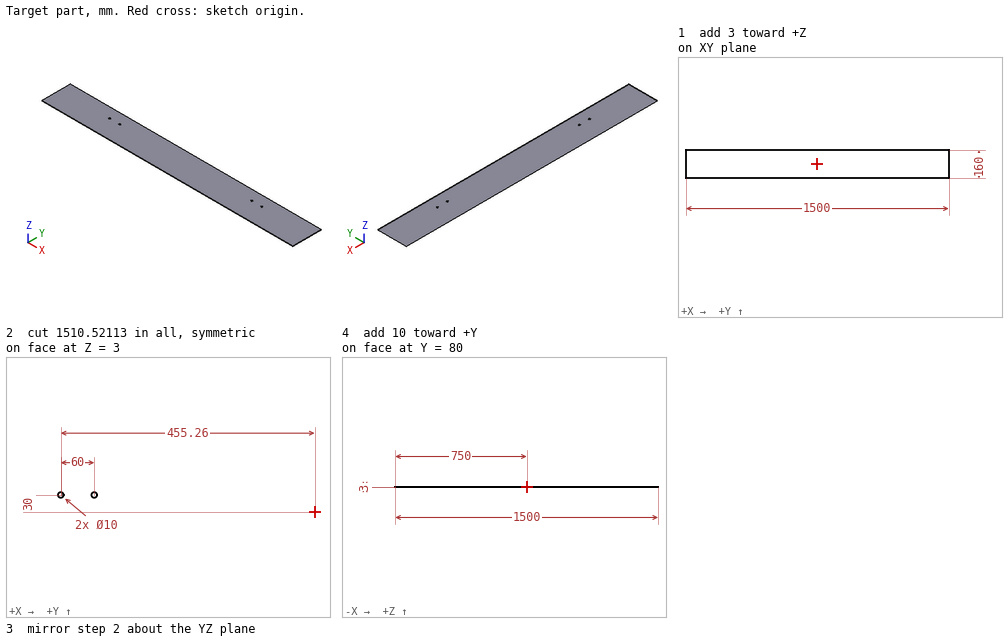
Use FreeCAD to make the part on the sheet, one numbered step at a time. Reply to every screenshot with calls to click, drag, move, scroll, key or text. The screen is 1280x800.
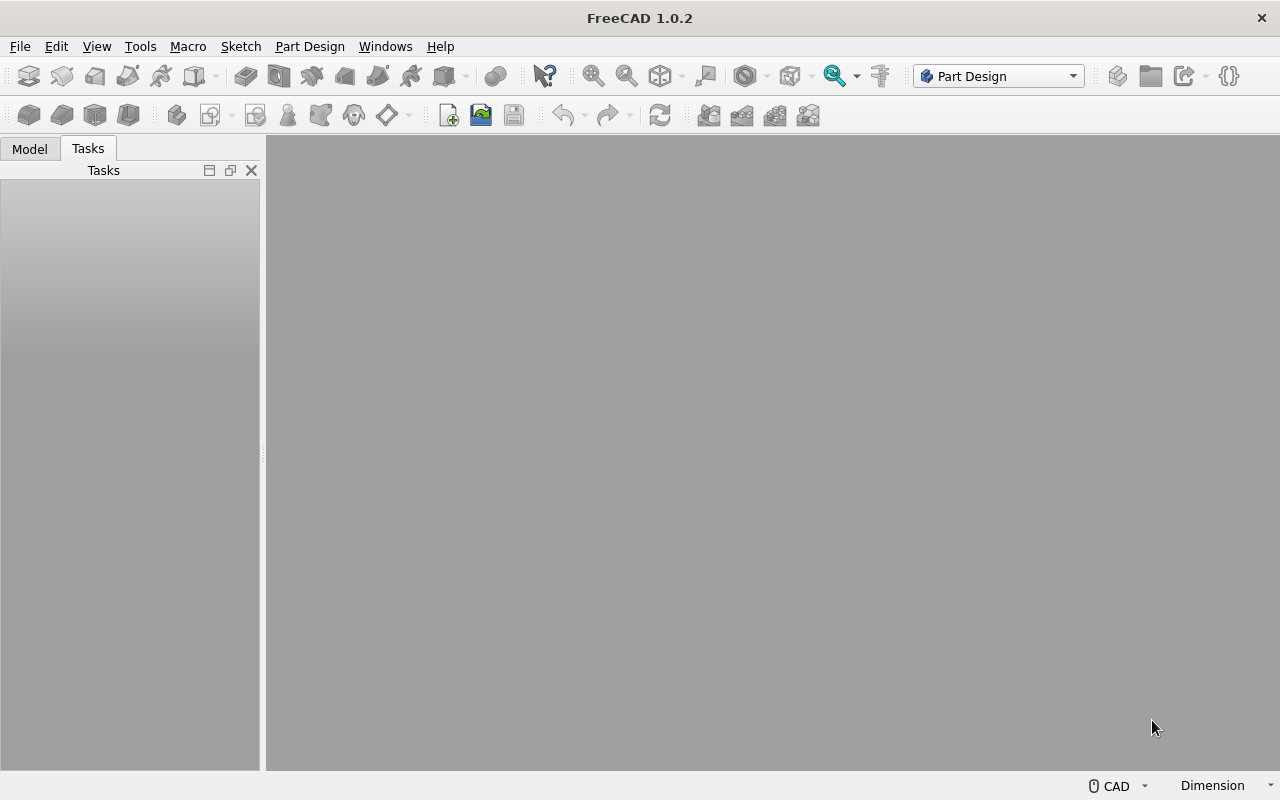
click(448, 116)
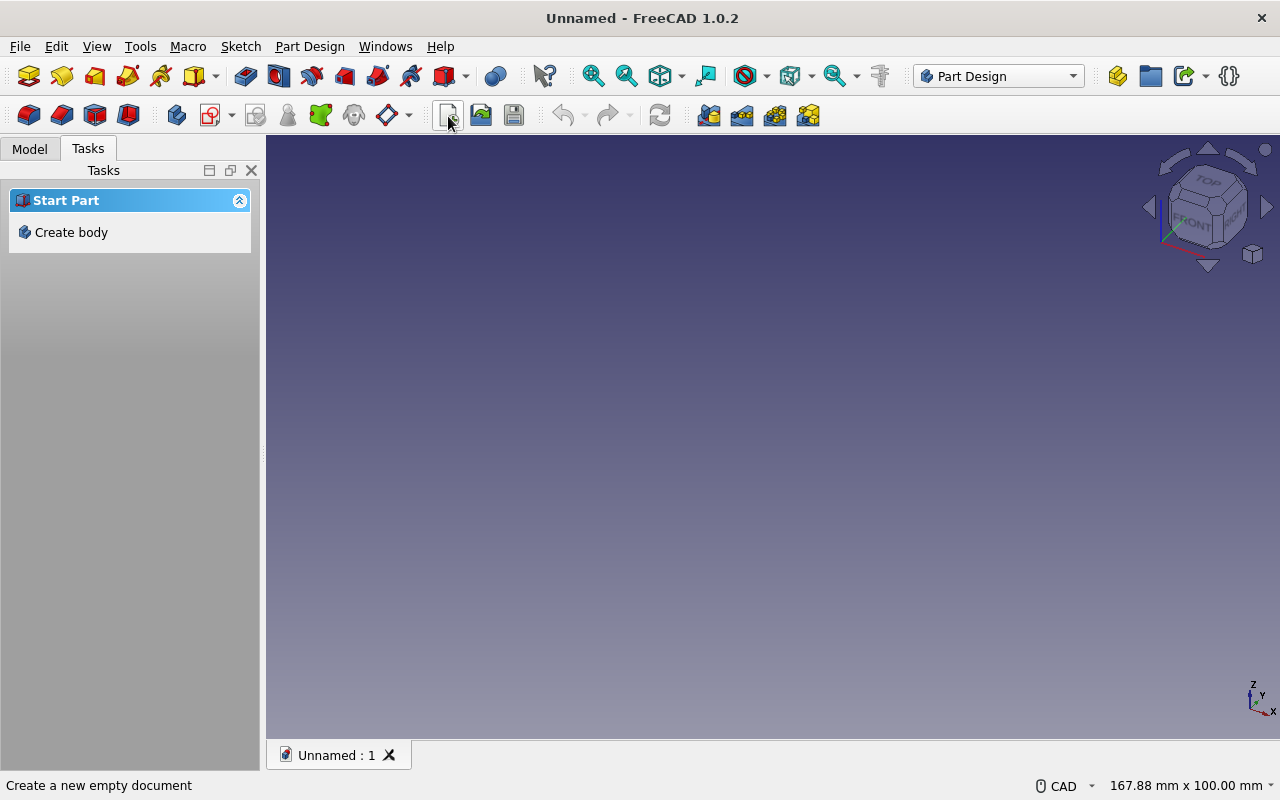
click(210, 116)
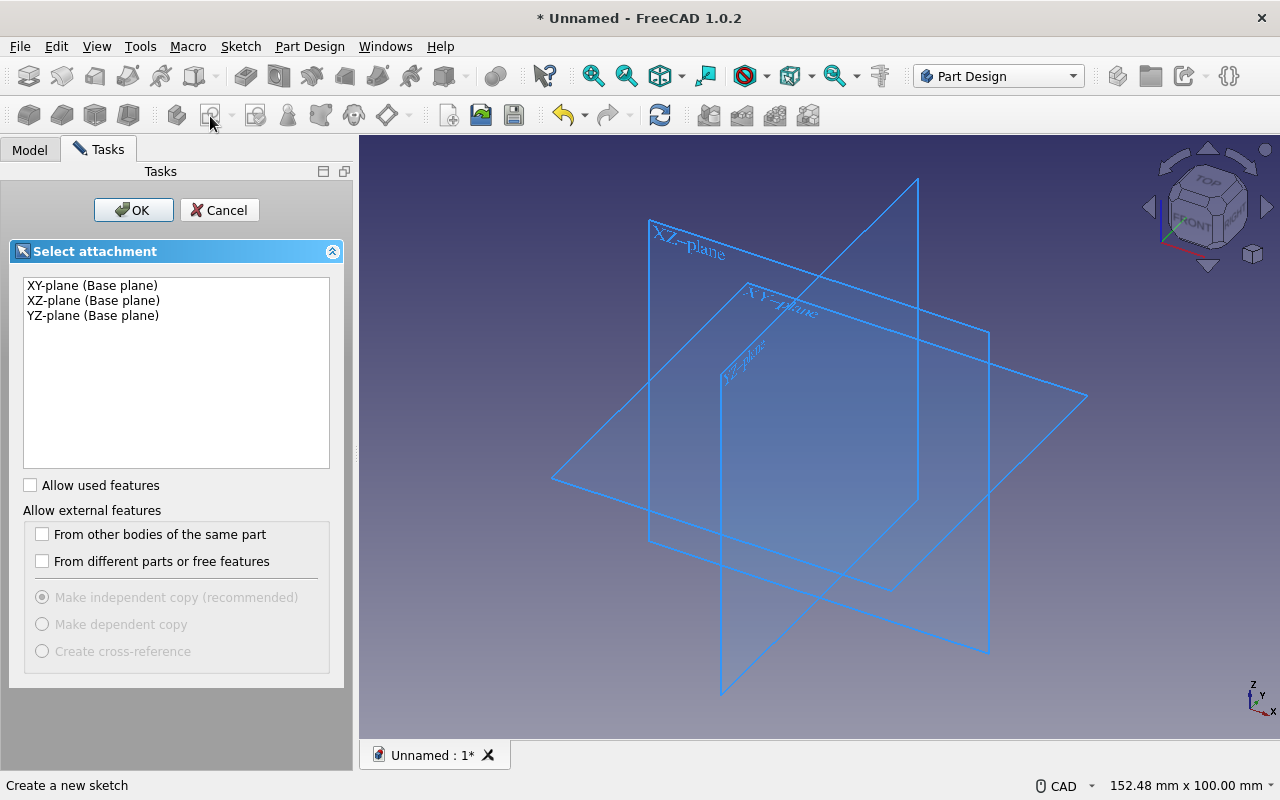
click(84, 286)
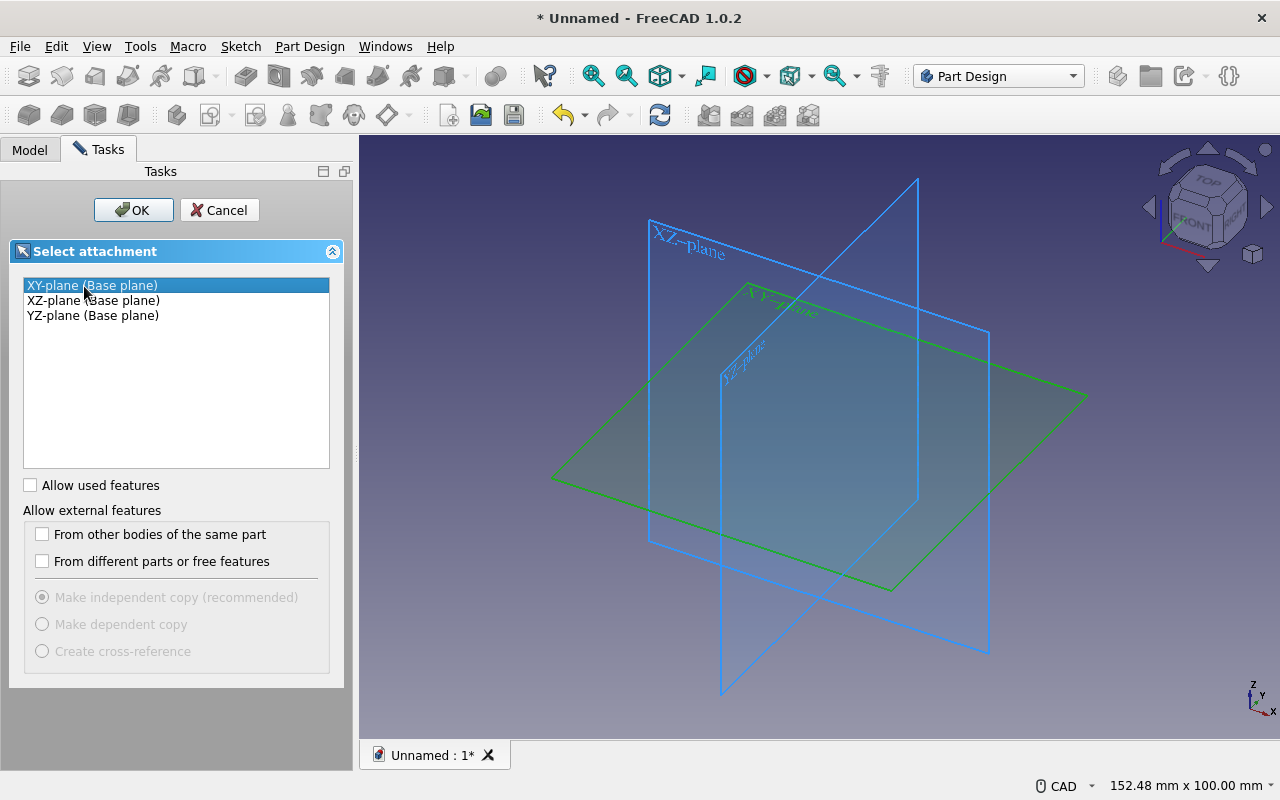
click(134, 210)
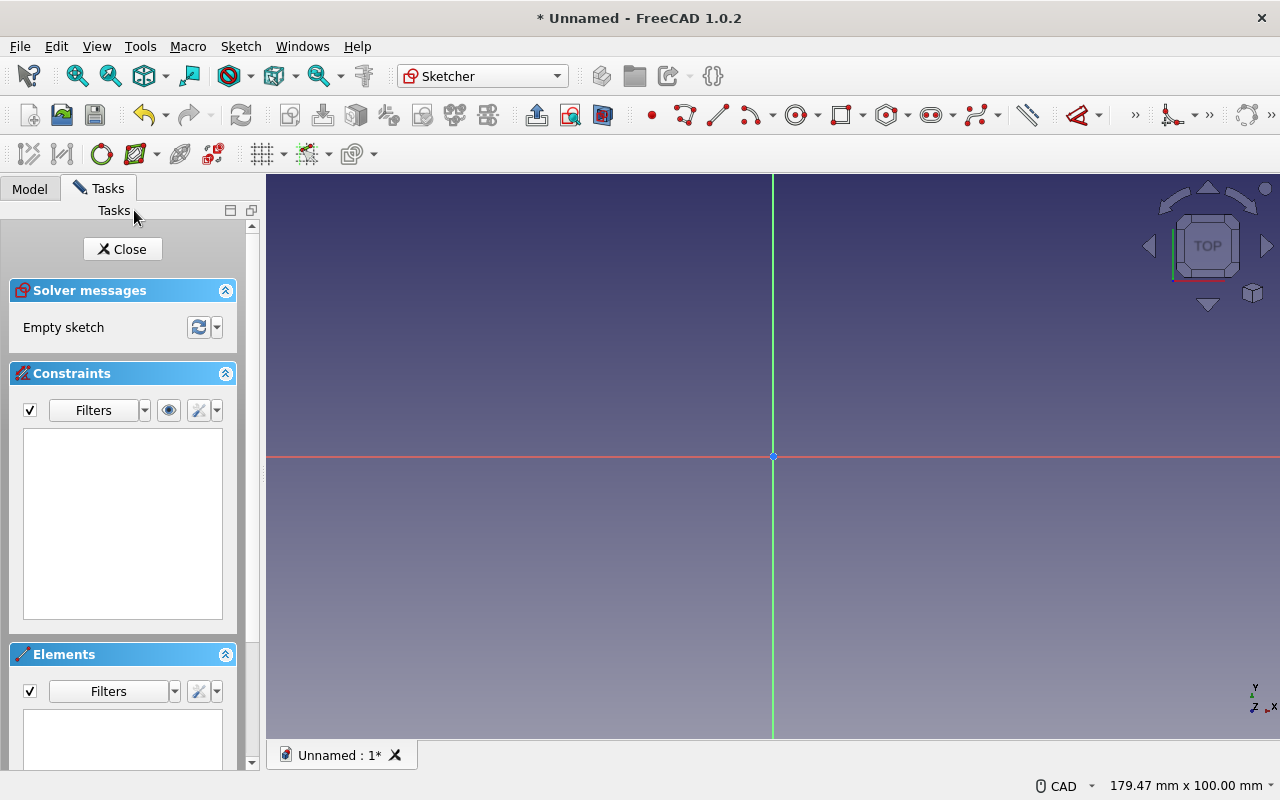
scroll(699, 456, down, 13)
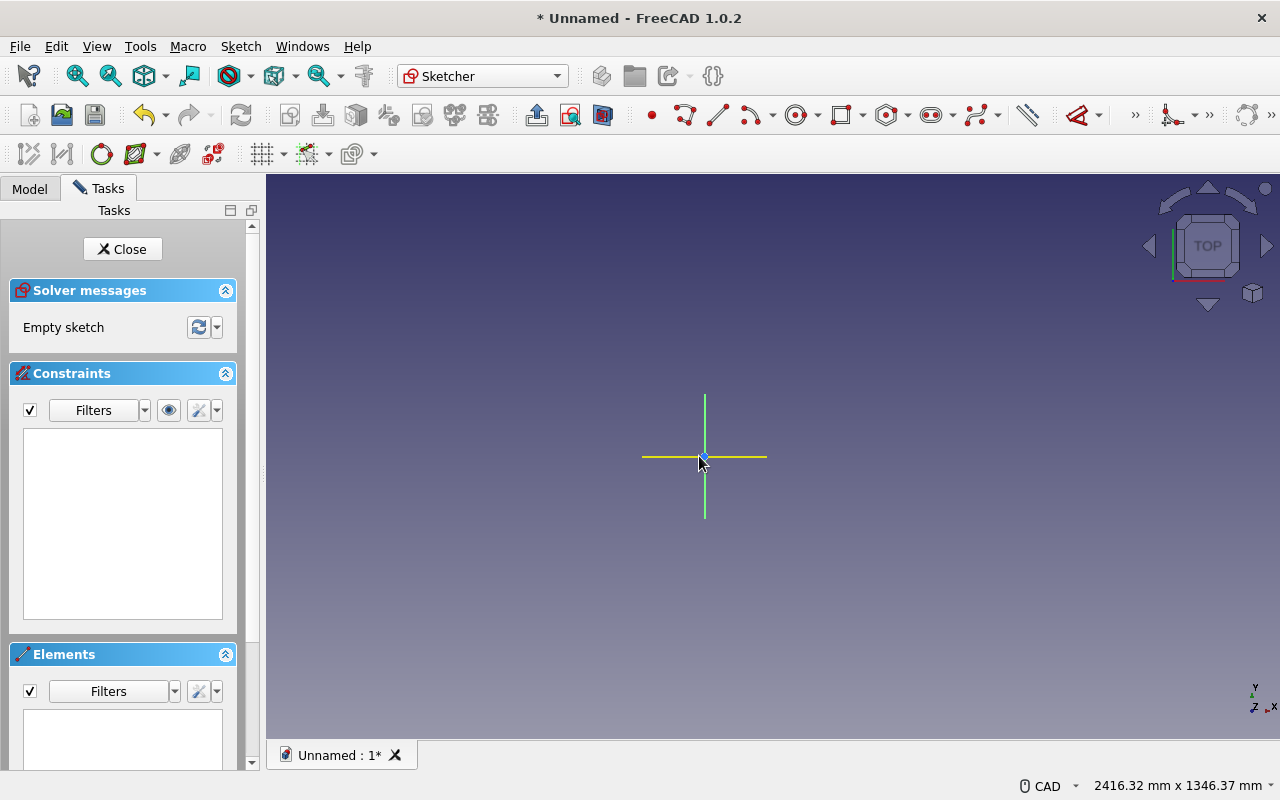
click(862, 116)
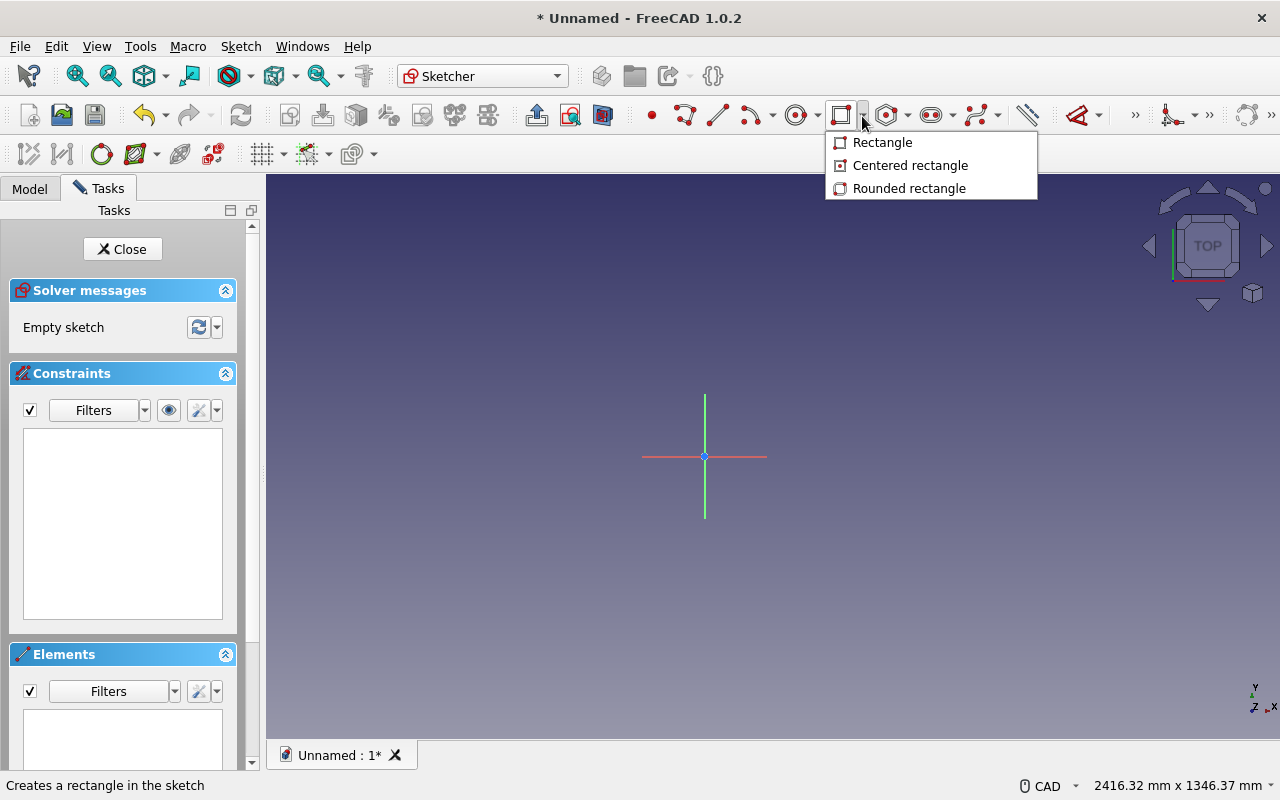
click(932, 166)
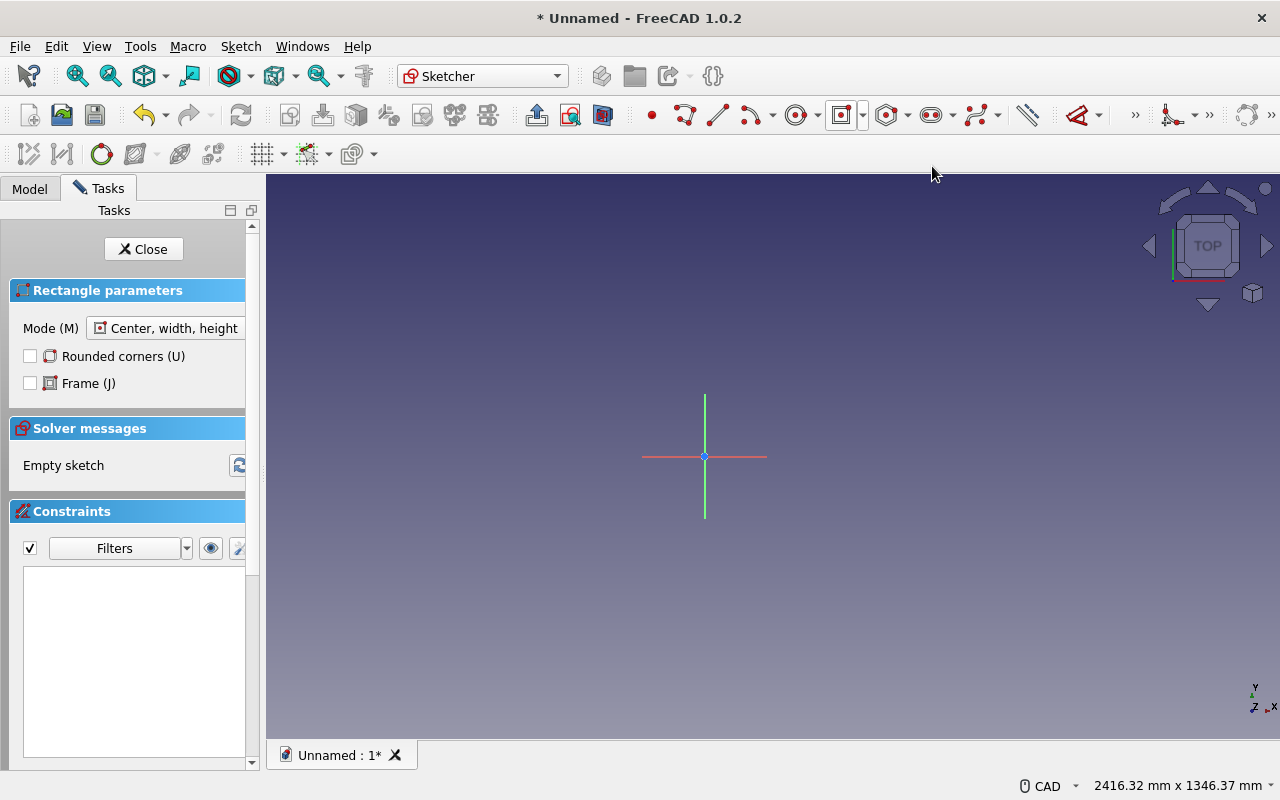
click(705, 456)
move(1020, 423)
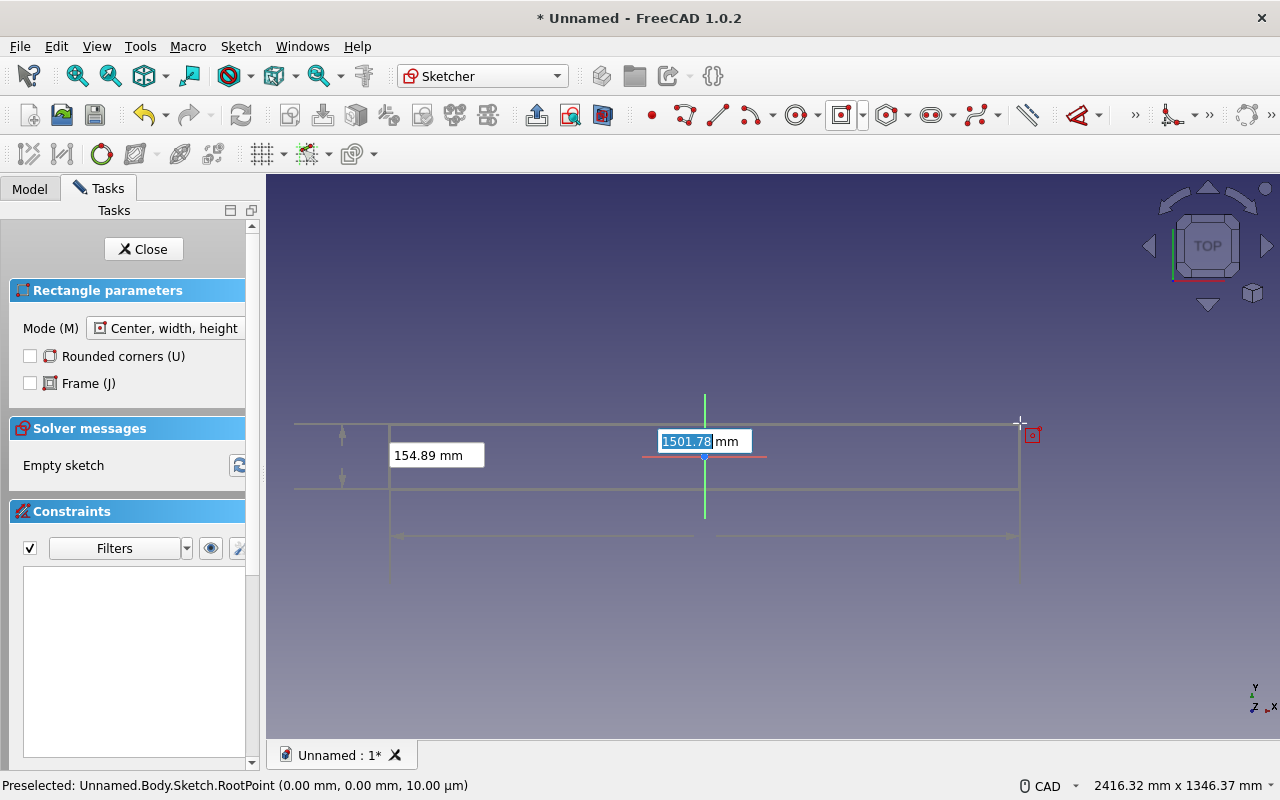
text(1500)
key(Tab)
text(160)
key(Return)
key(Escape)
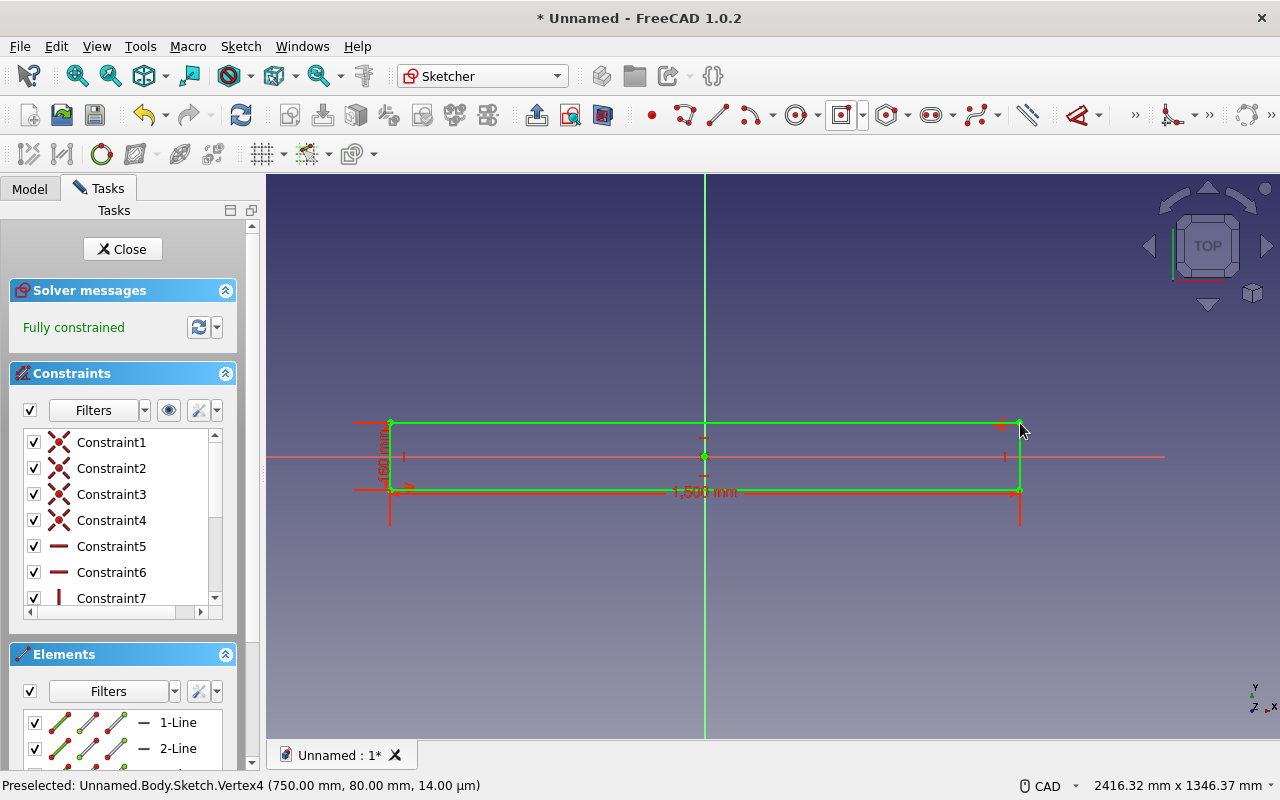
click(123, 249)